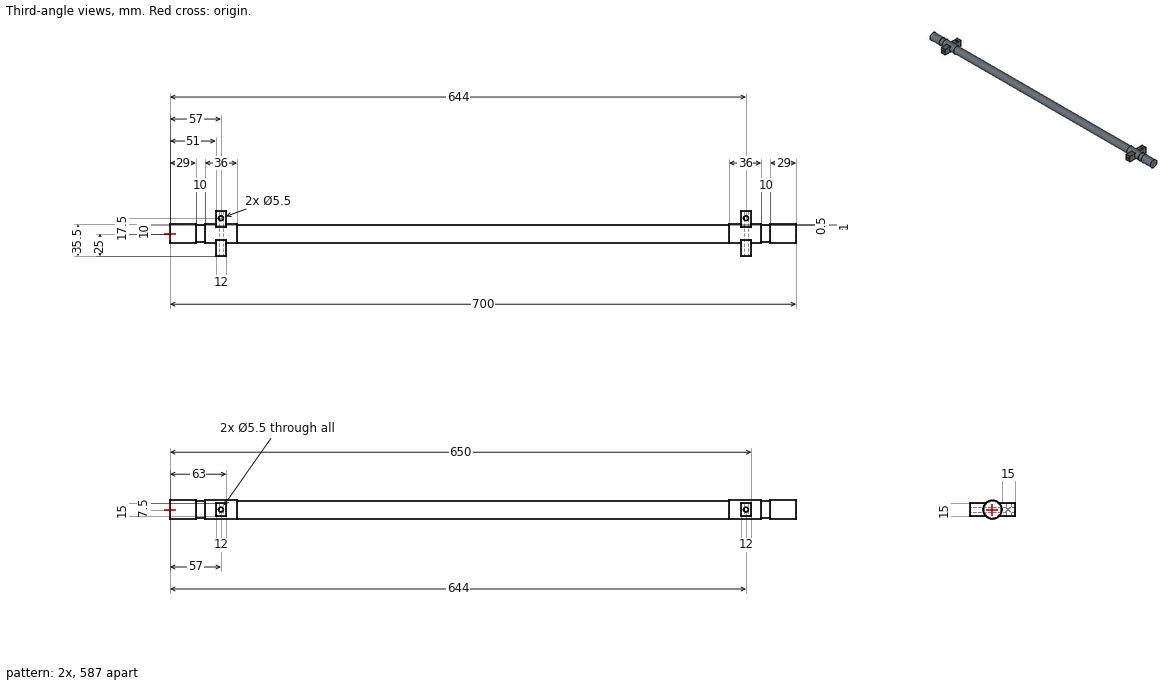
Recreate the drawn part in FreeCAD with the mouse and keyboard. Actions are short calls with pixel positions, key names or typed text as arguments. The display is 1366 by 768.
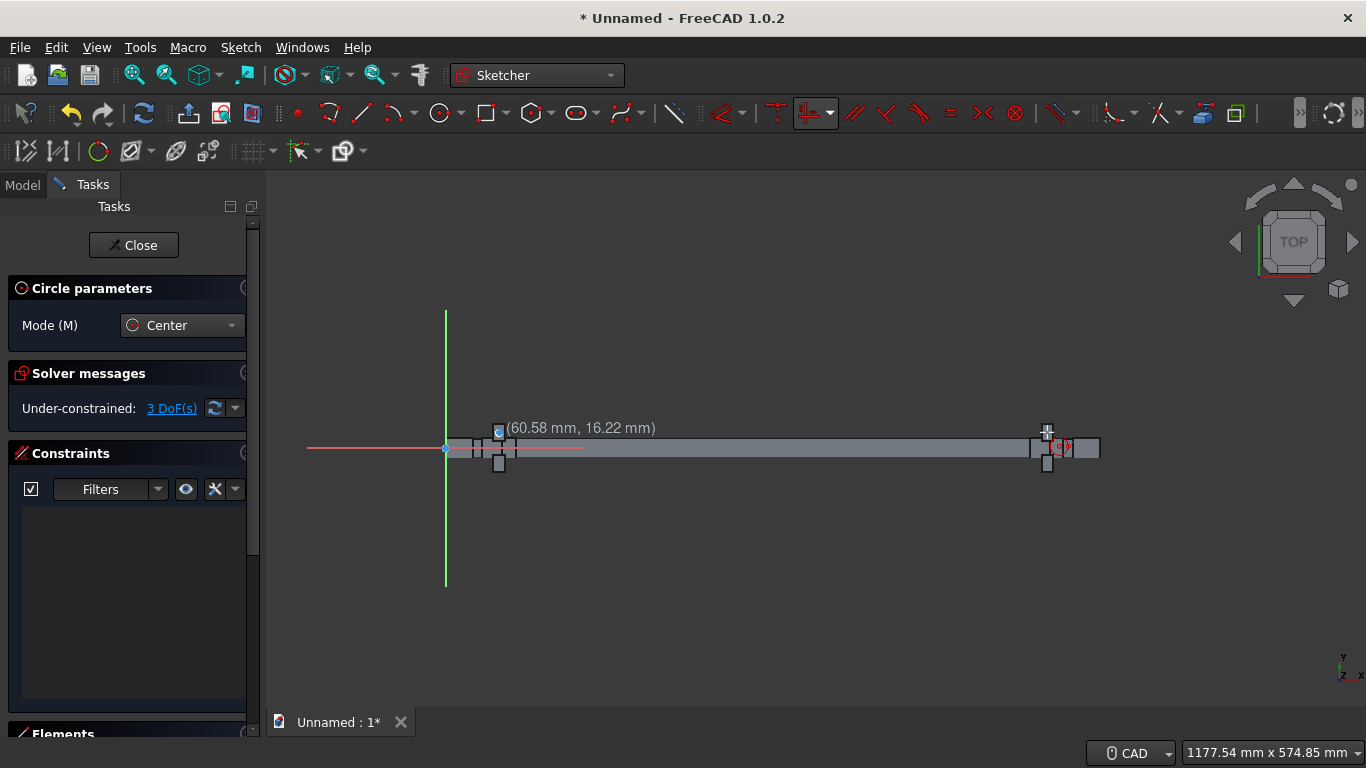
click(1047, 432)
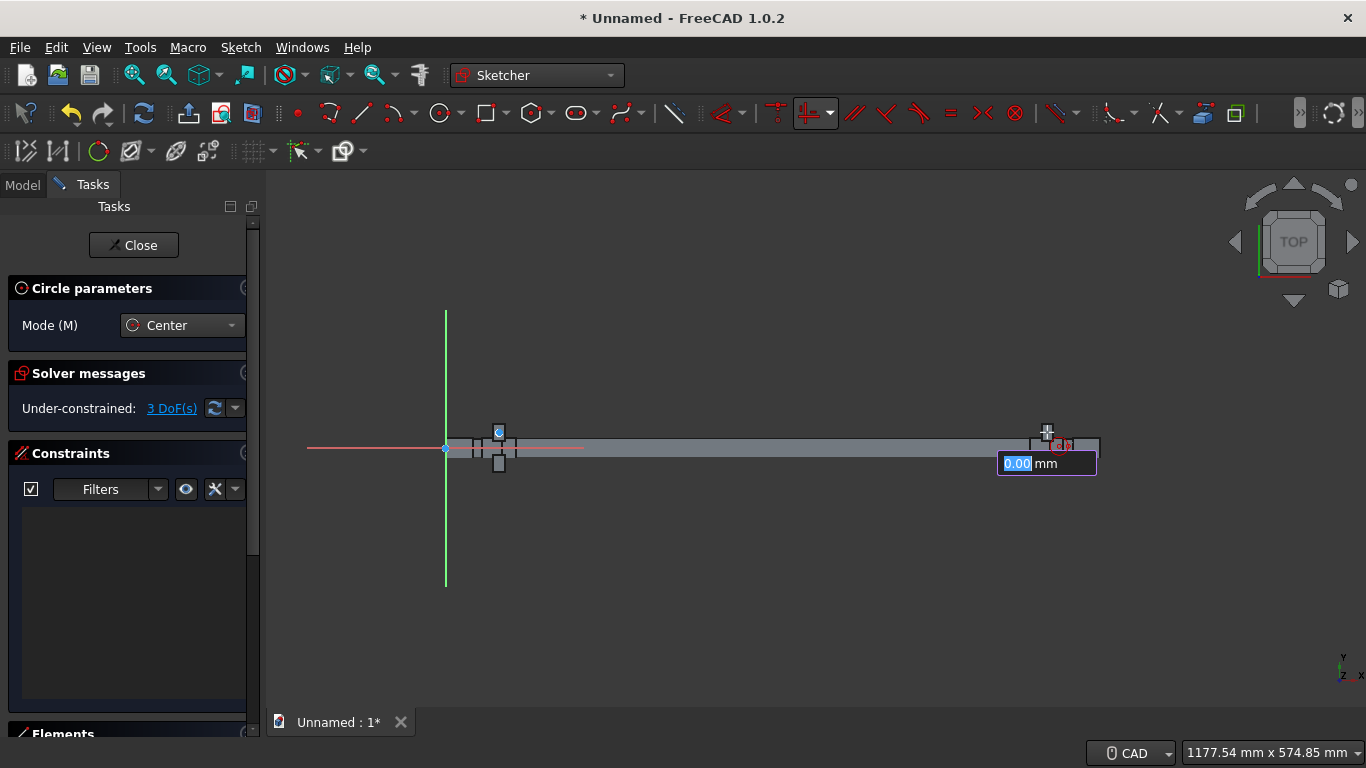
scroll(1049, 430, up, 10)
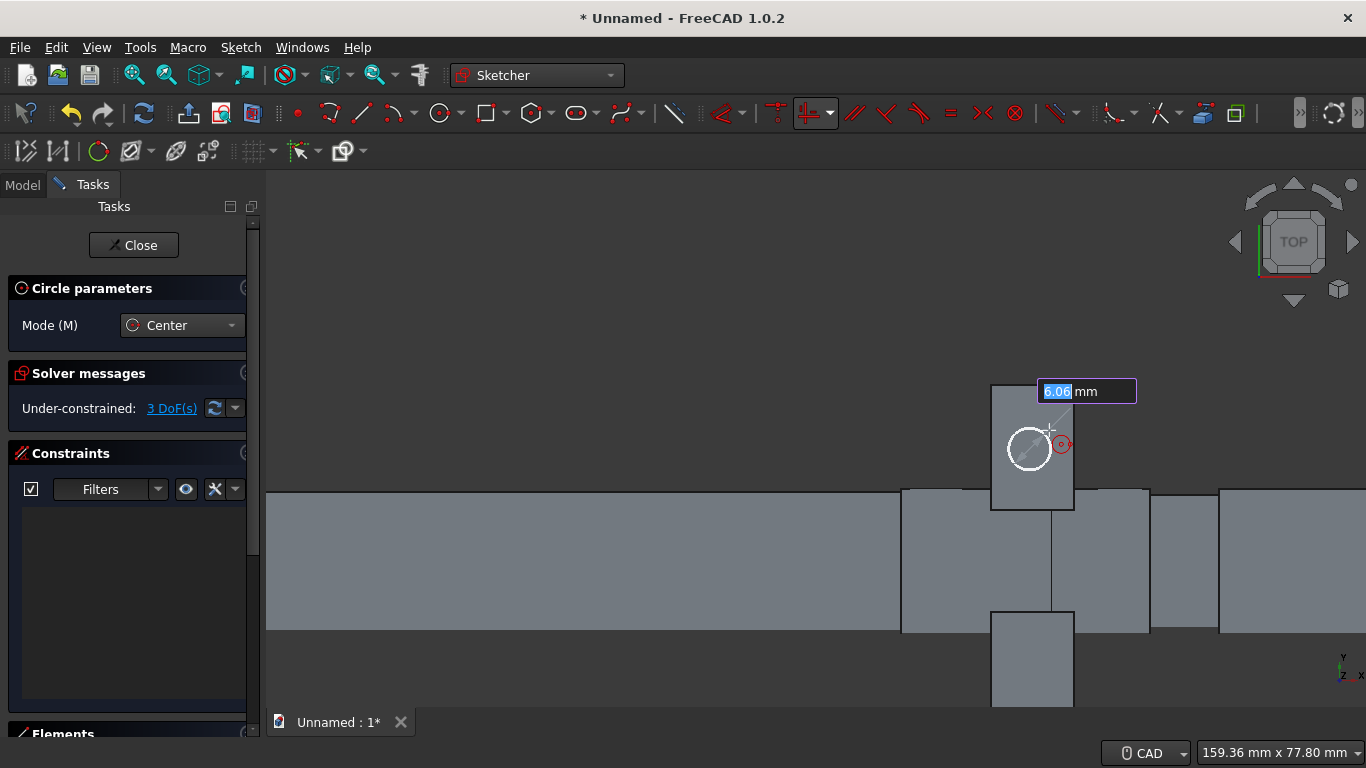
click(1046, 427)
key(Escape)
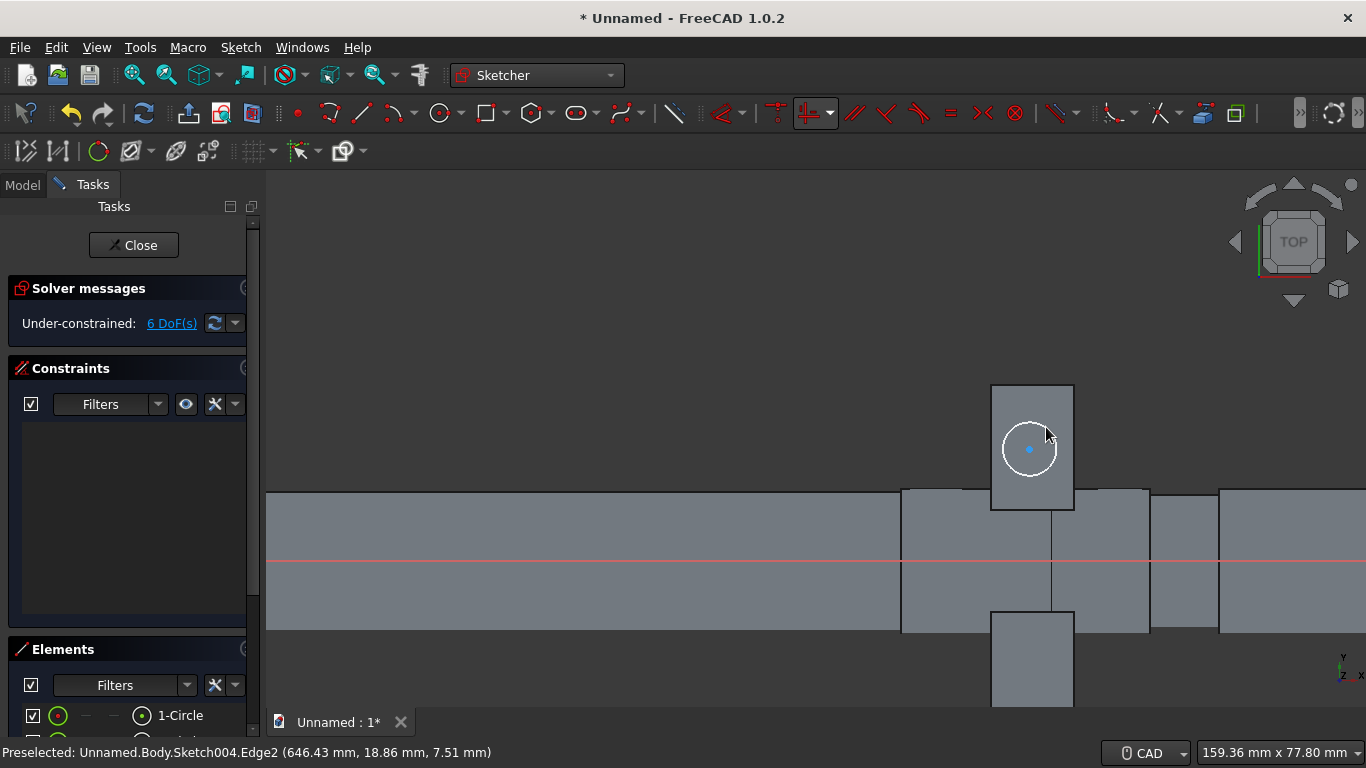
scroll(1049, 430, down, 10)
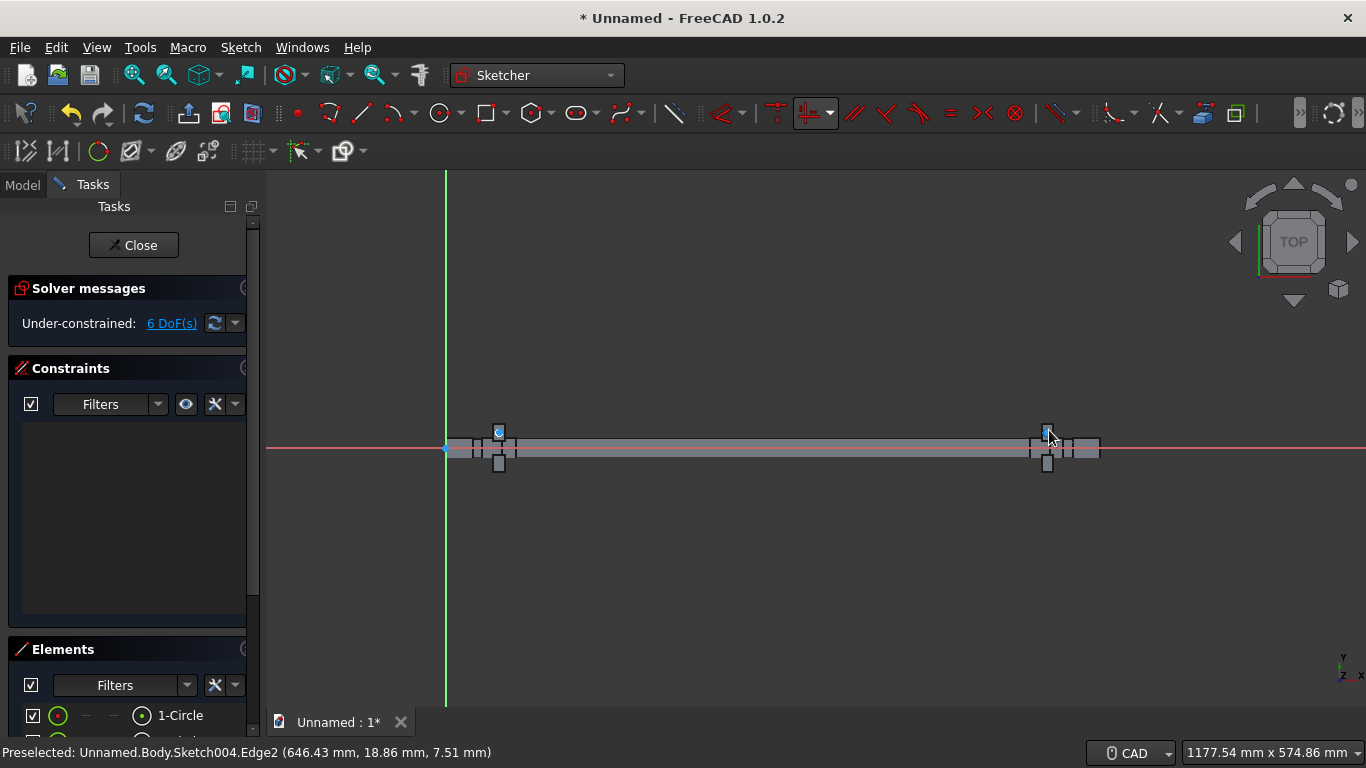
scroll(501, 431, up, 8)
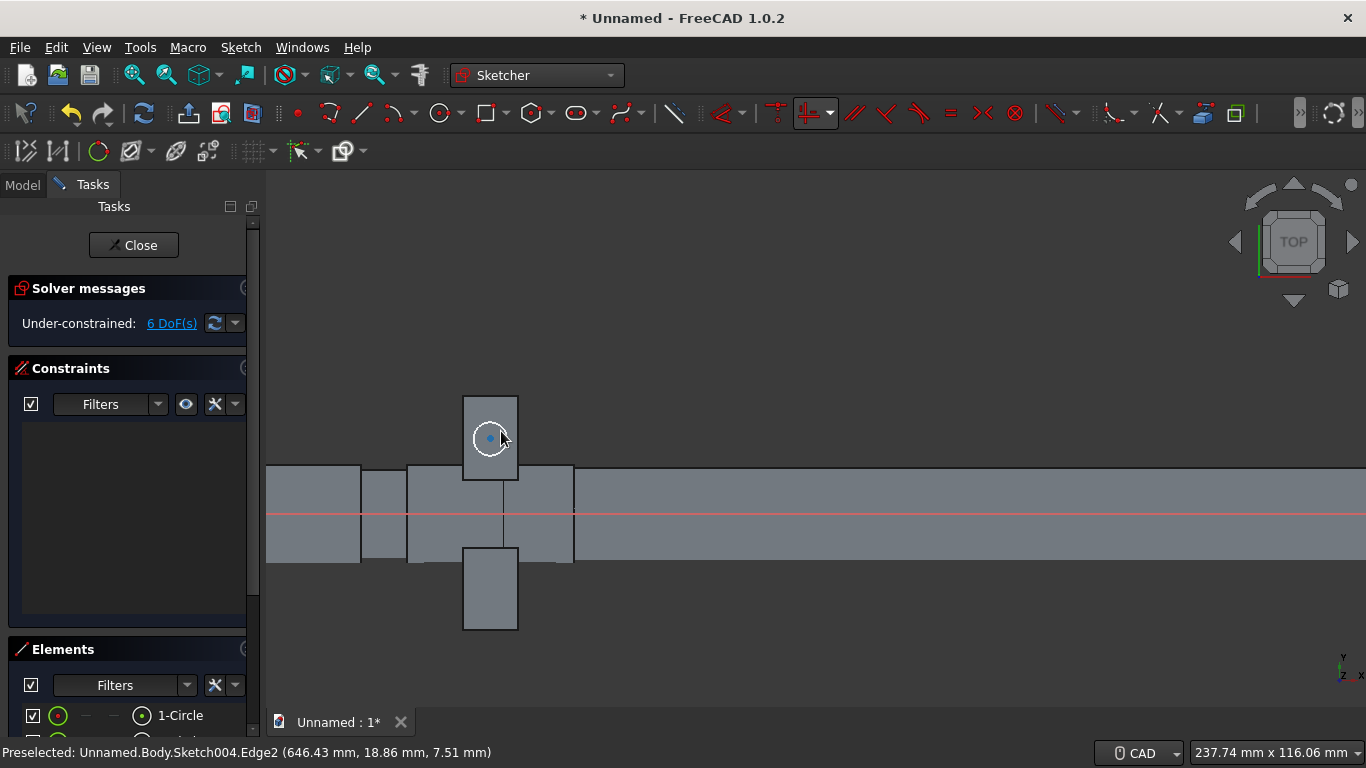
click(502, 427)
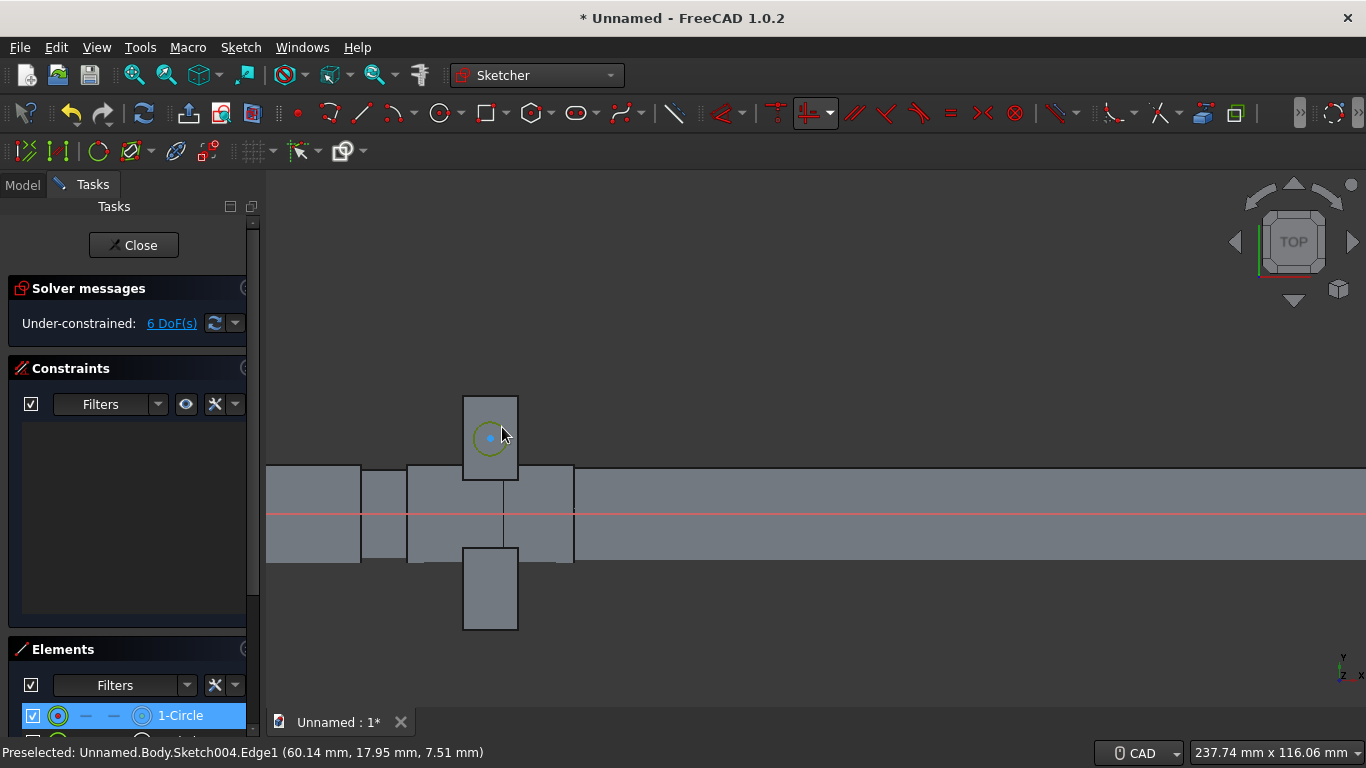
scroll(501, 431, down, 8)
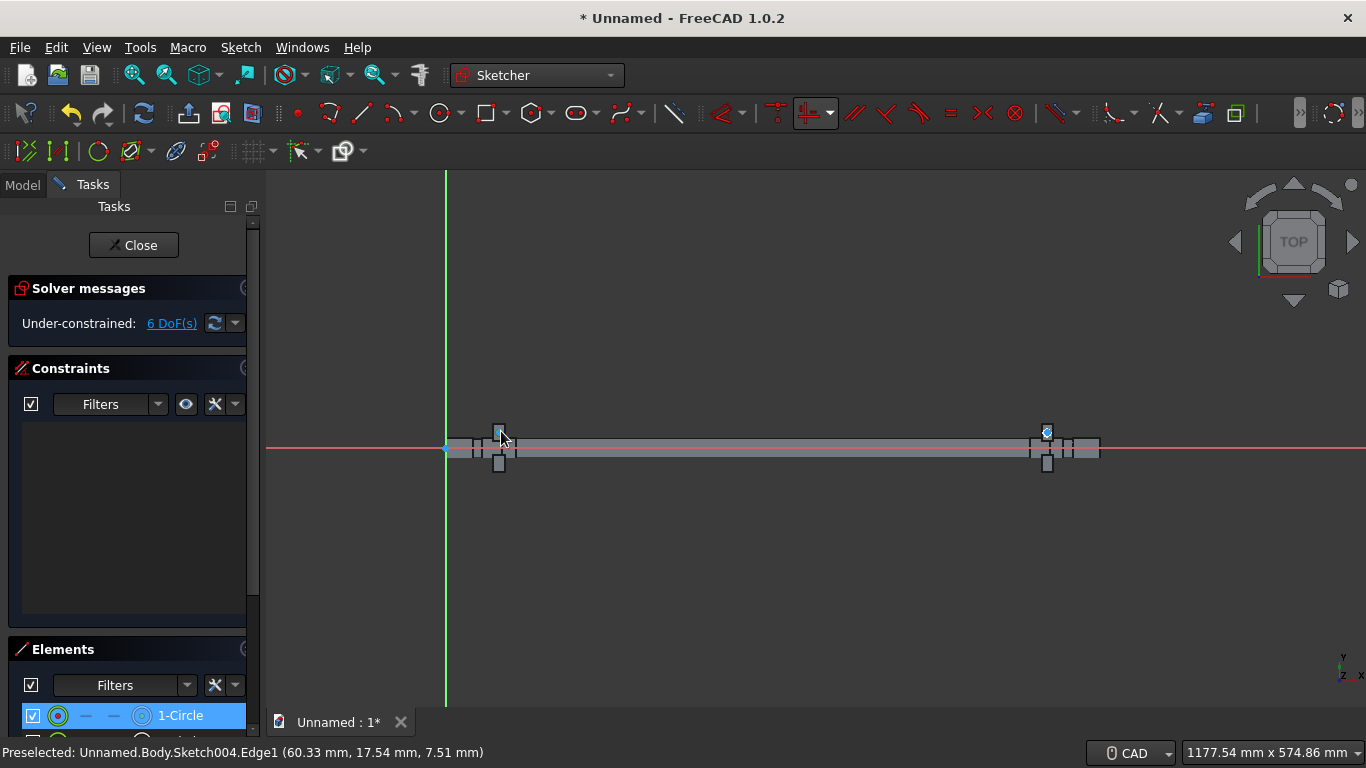
scroll(1050, 430, up, 7)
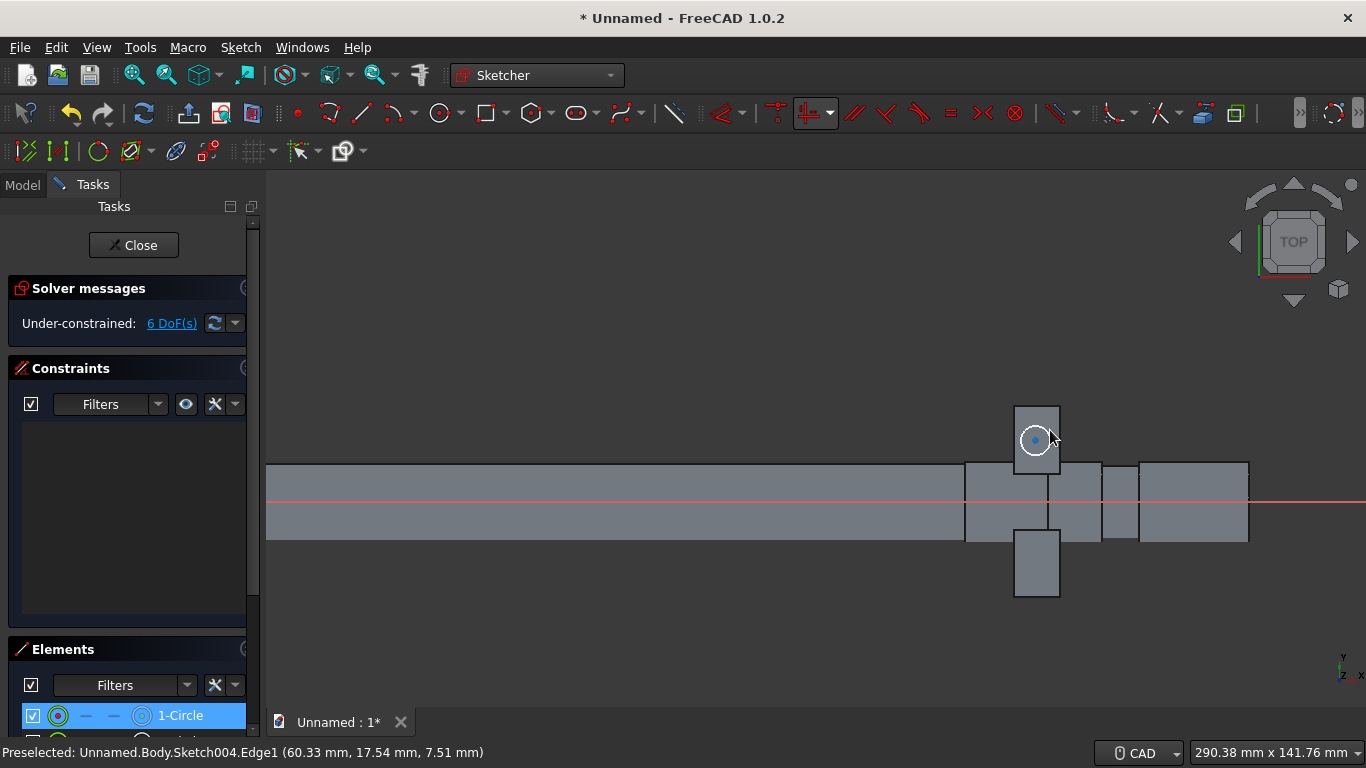
click(1046, 430)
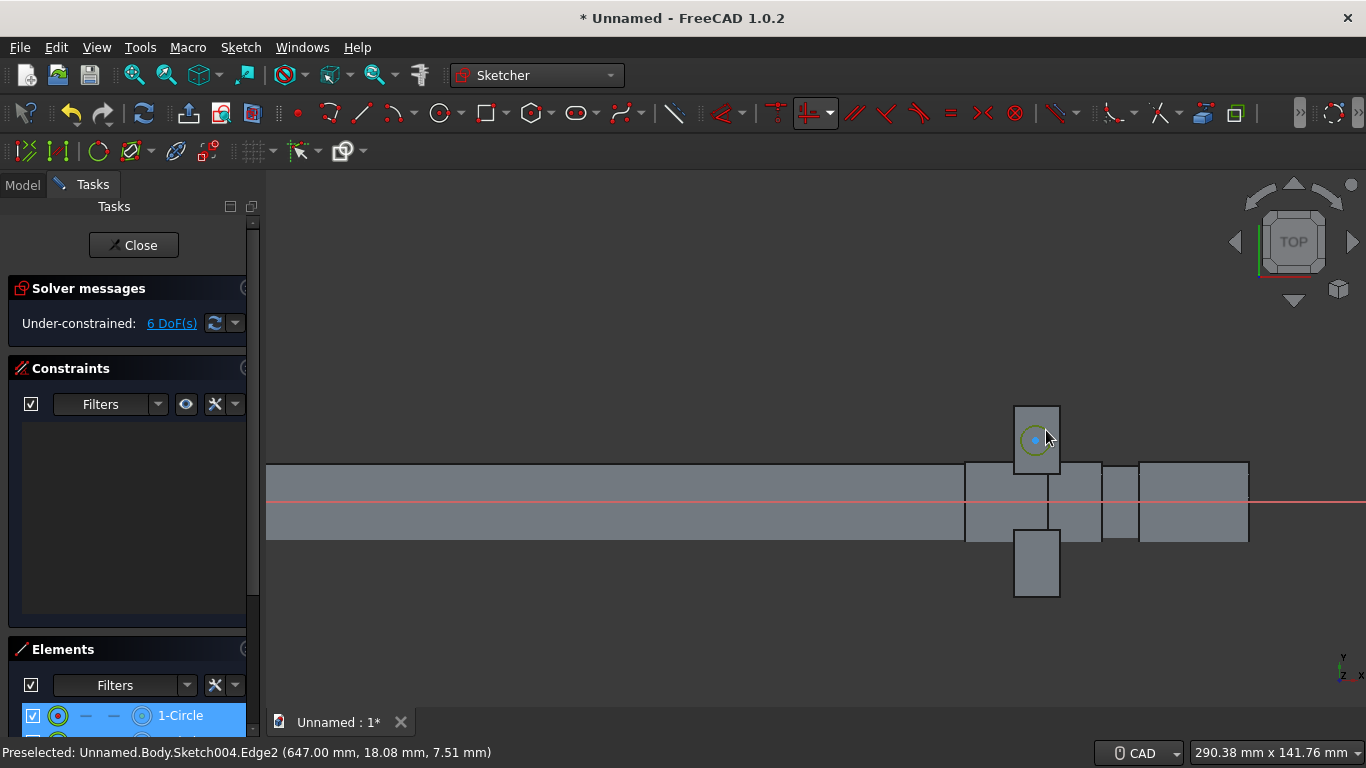
click(952, 114)